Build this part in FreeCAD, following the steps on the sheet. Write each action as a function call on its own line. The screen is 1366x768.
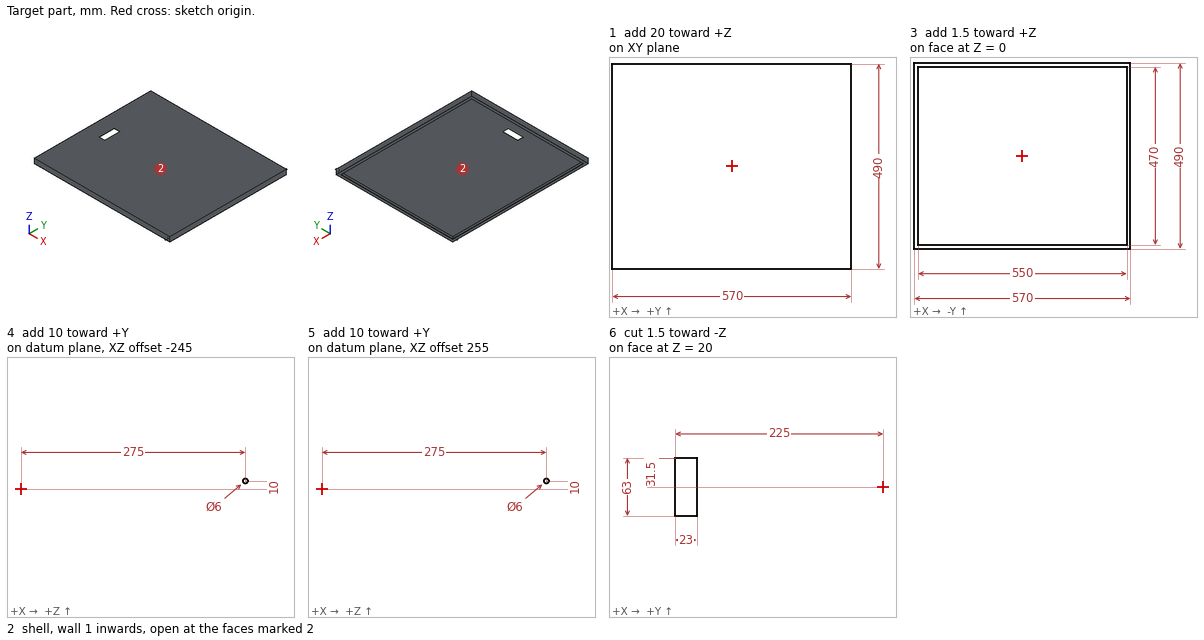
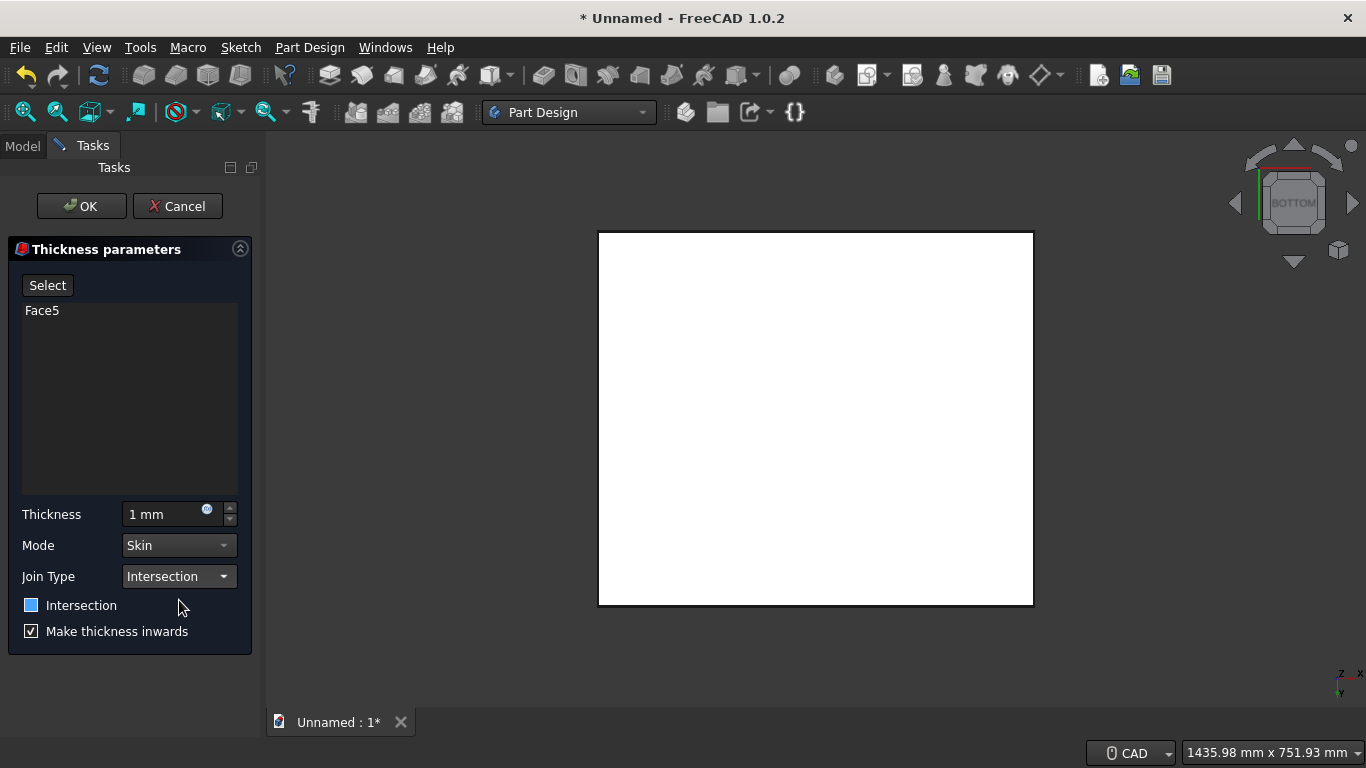
click(82, 206)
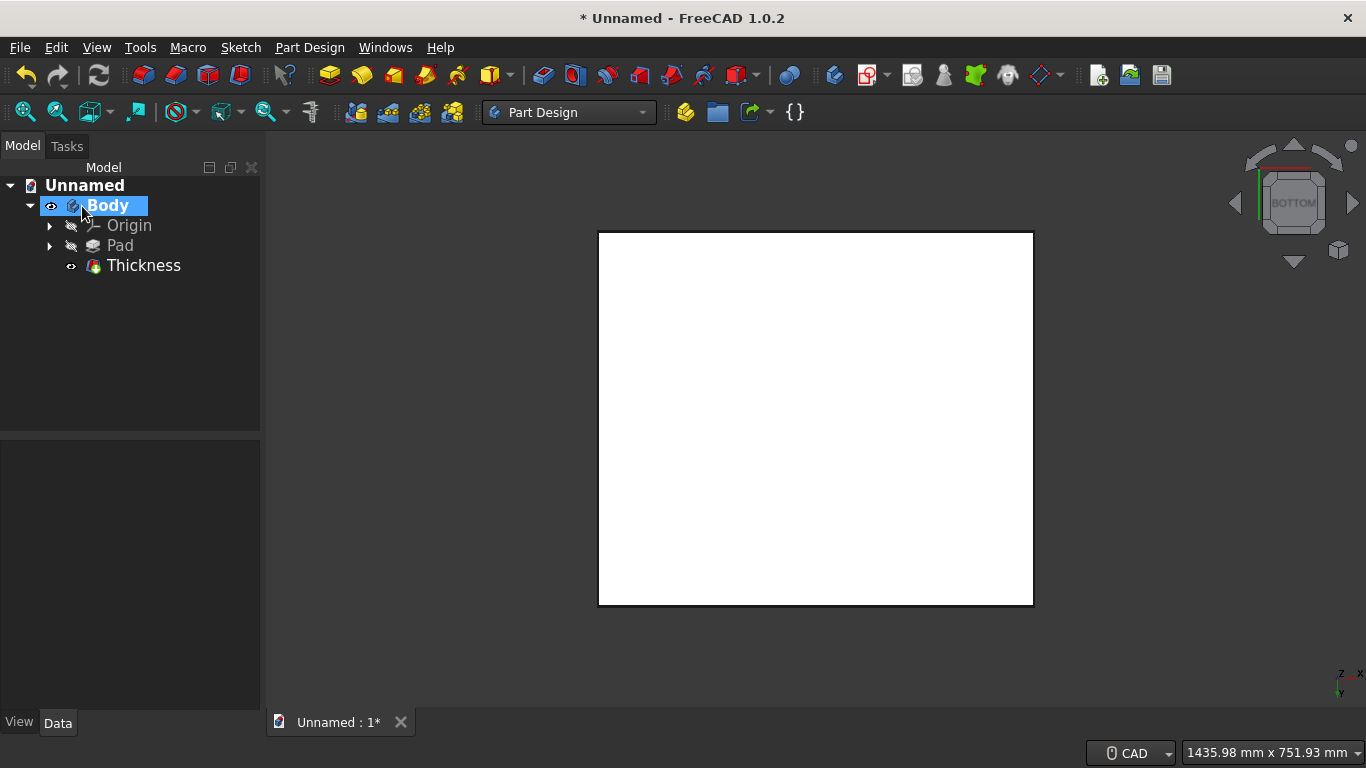
scroll(889, 605, up, 15)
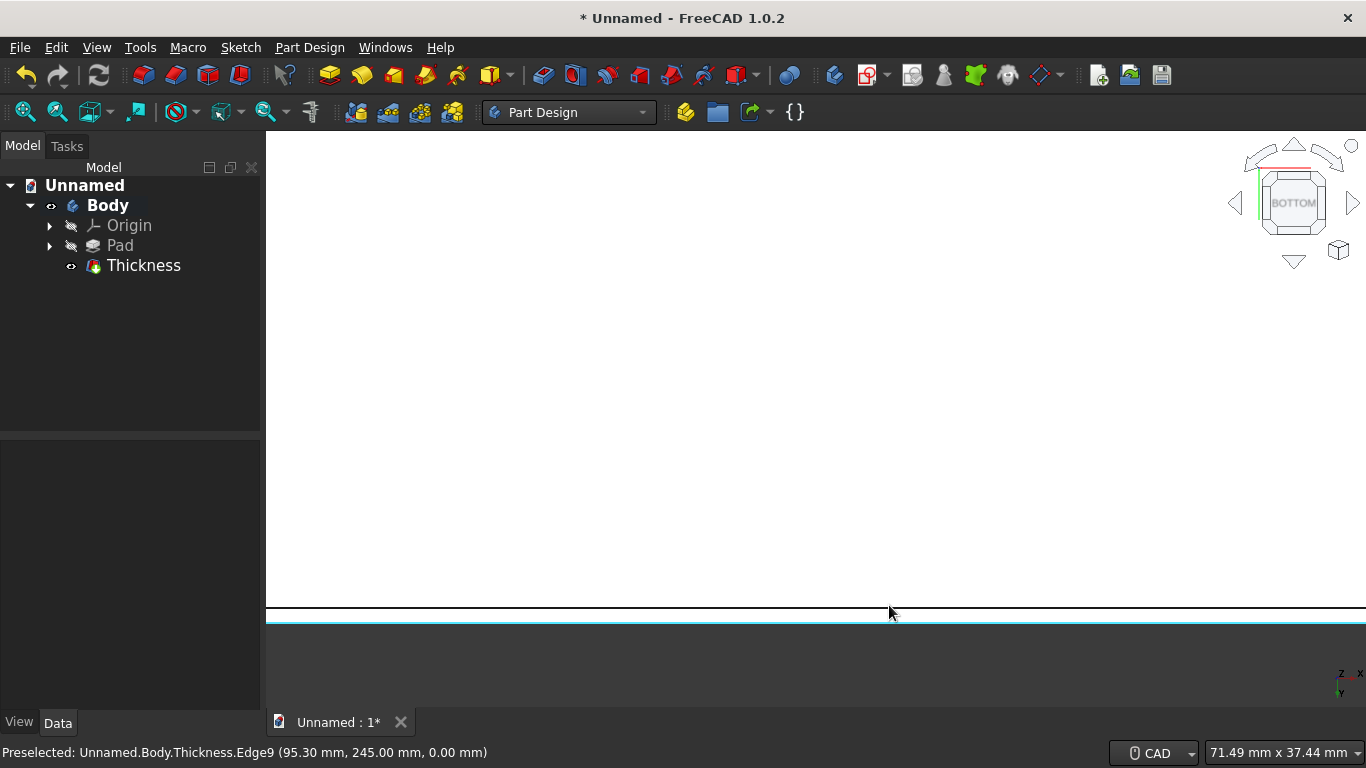
scroll(874, 612, up, 5)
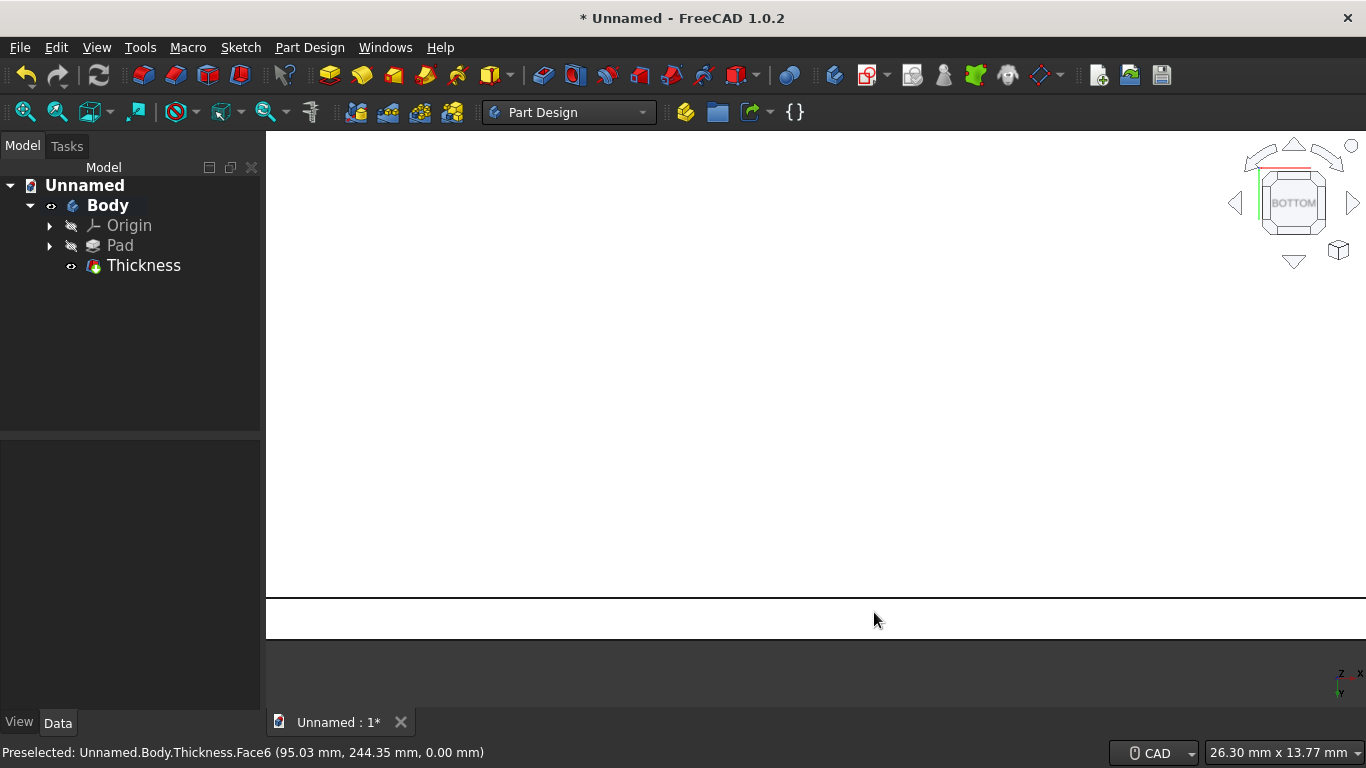
click(872, 611)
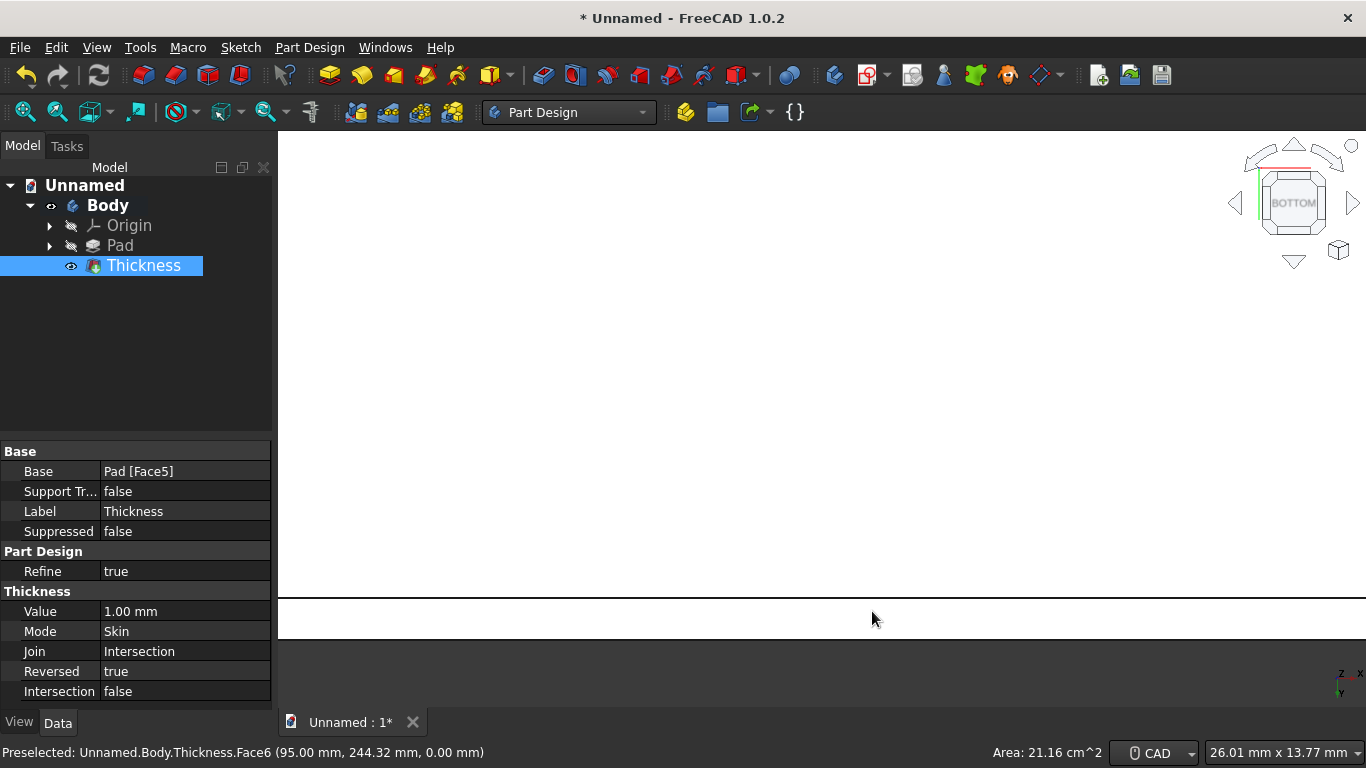
click(868, 76)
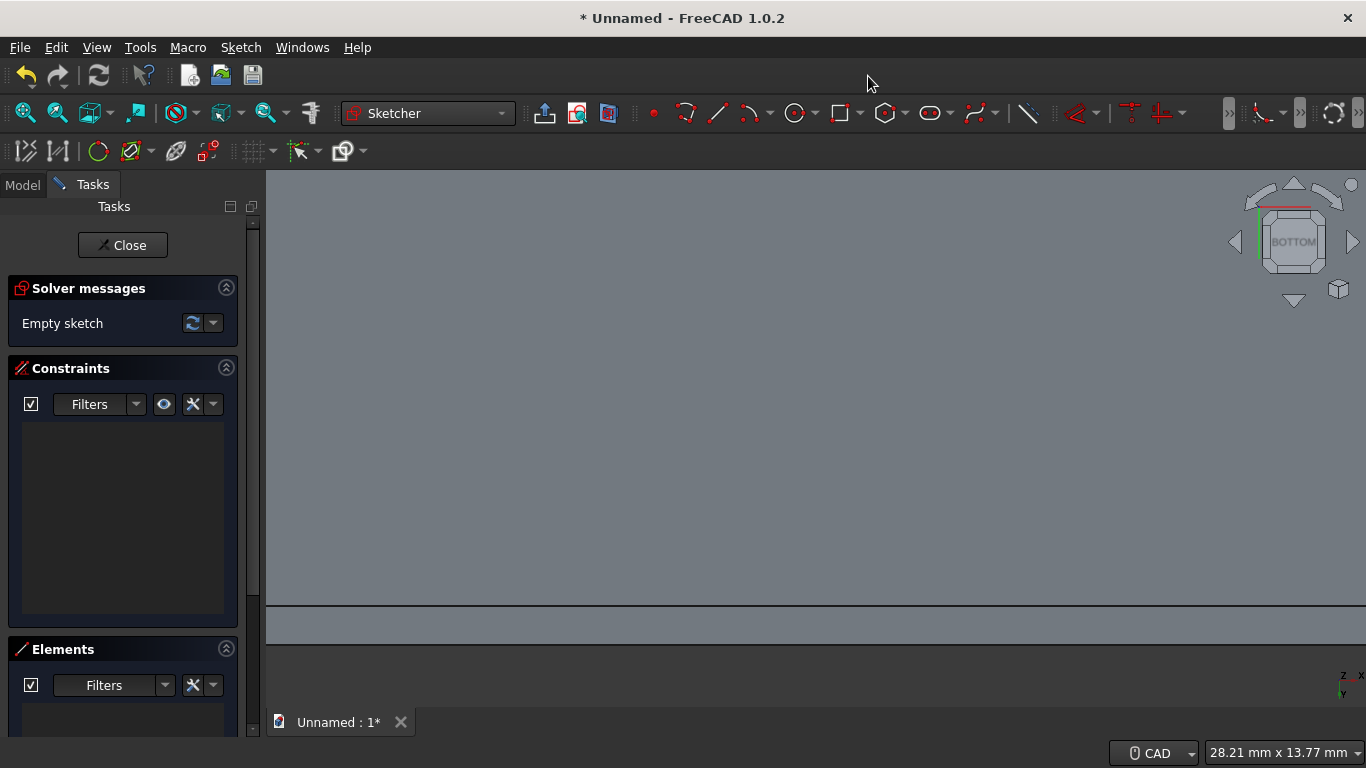
scroll(748, 438, down, 15)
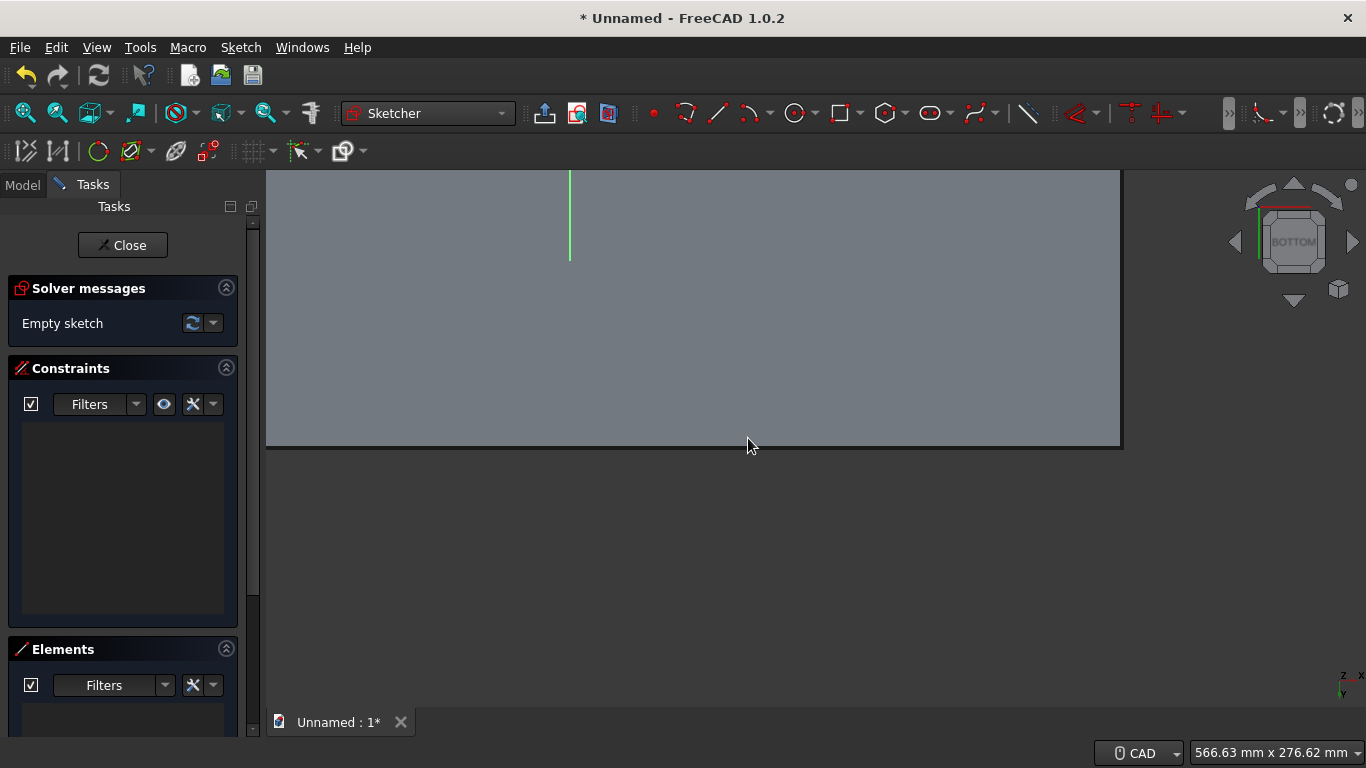
scroll(851, 679, down, 5)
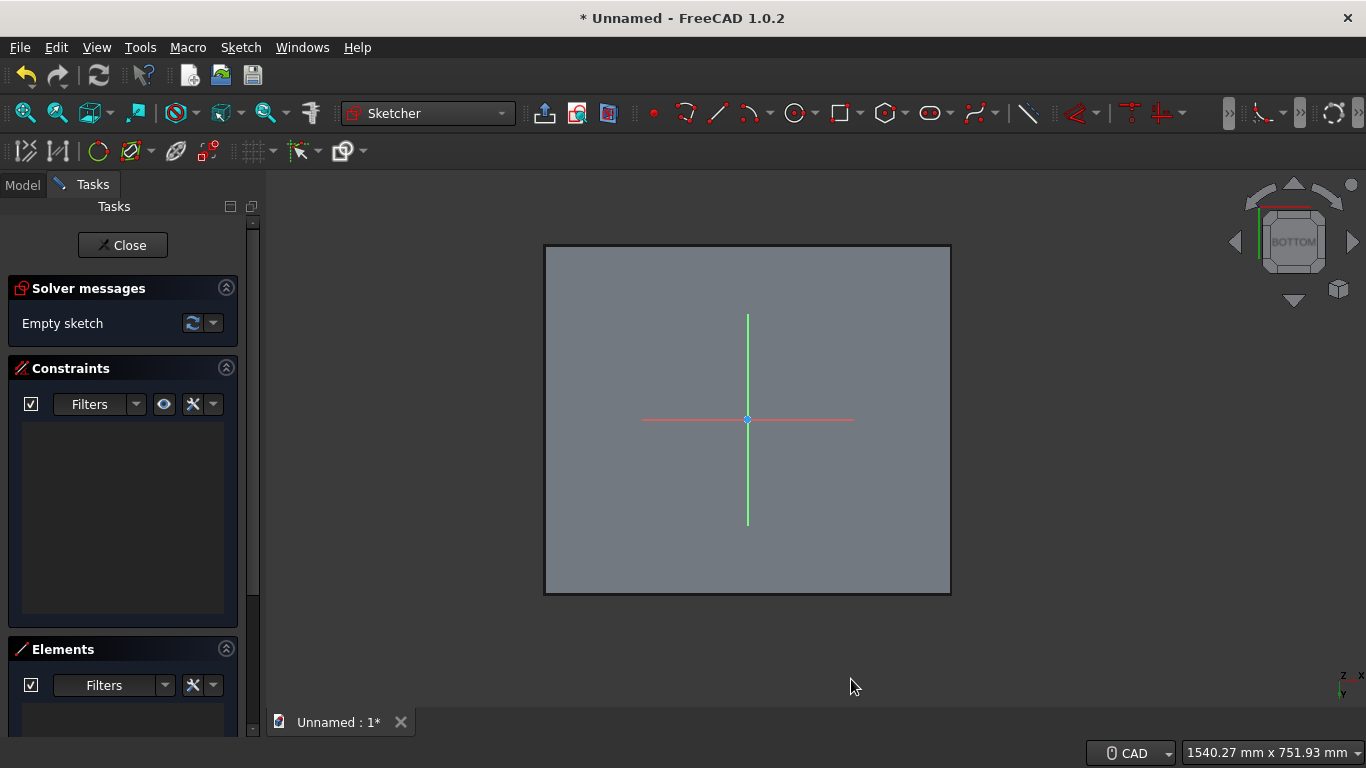
key(g)
key(v)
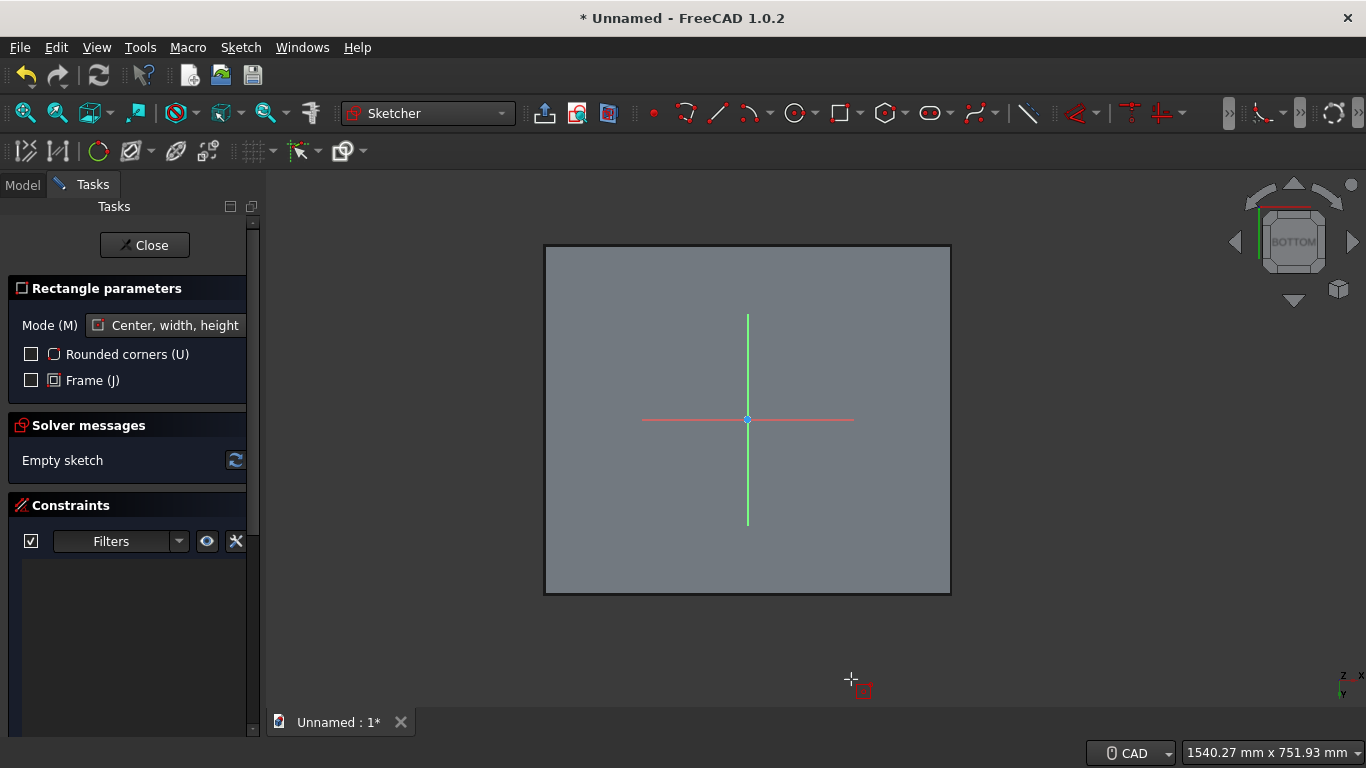
click(748, 420)
click(951, 245)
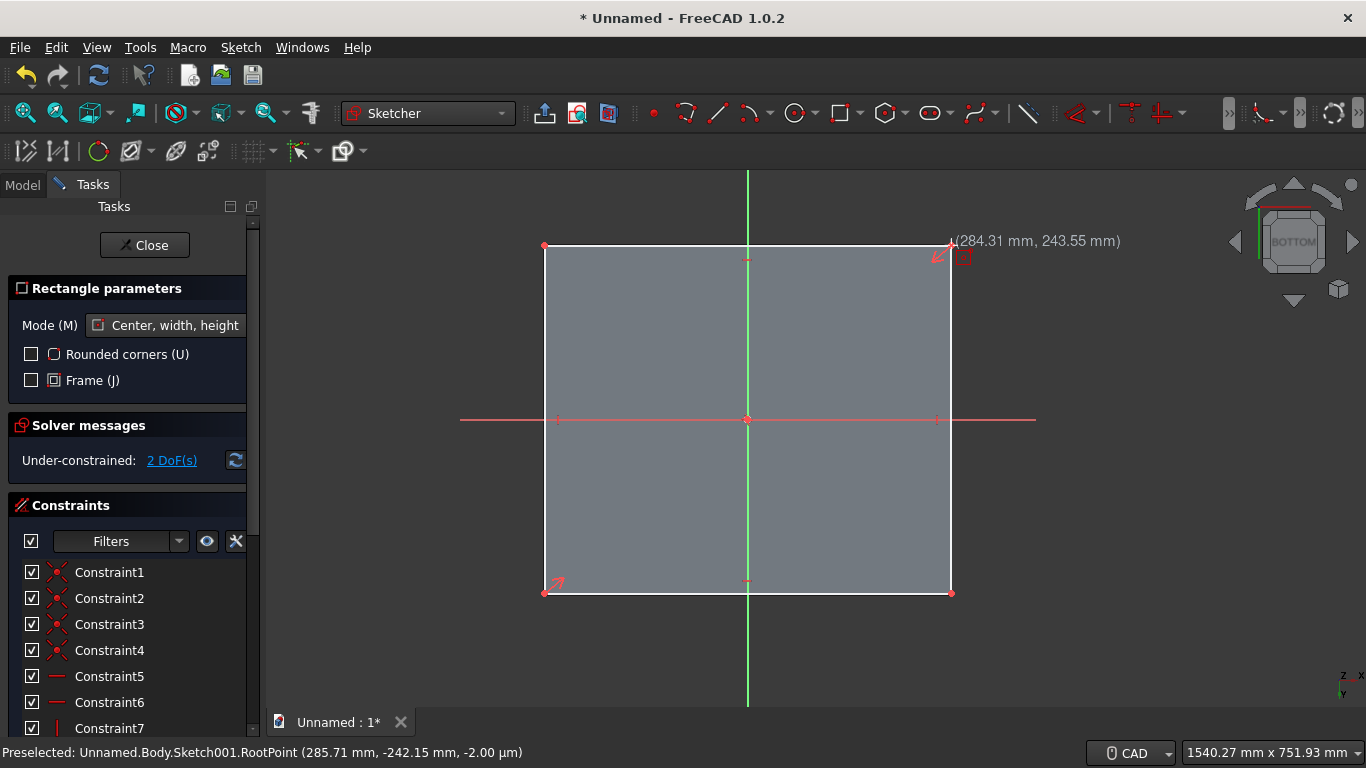
click(748, 420)